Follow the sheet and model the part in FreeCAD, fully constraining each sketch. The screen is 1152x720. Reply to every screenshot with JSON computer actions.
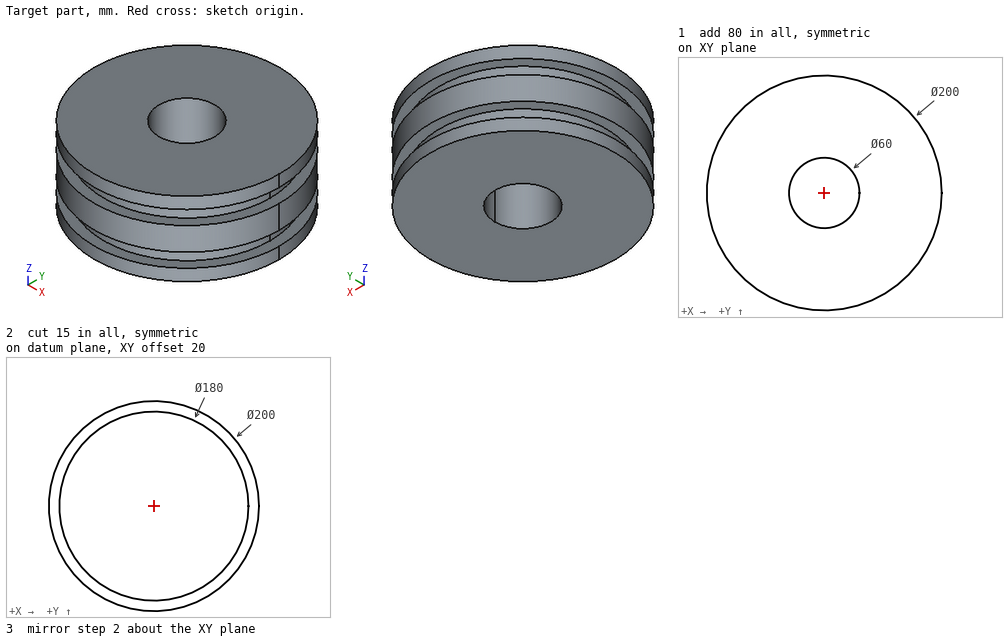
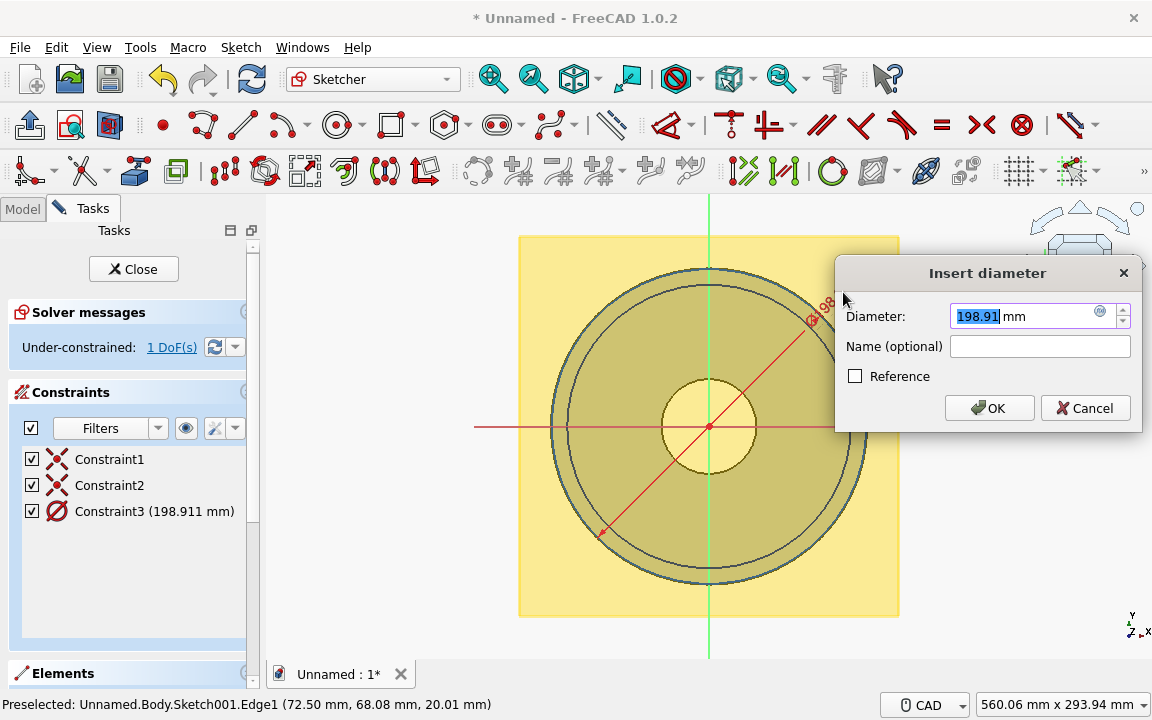
{"action": "type", "text": "200"}
{"action": "key", "text": "Return"}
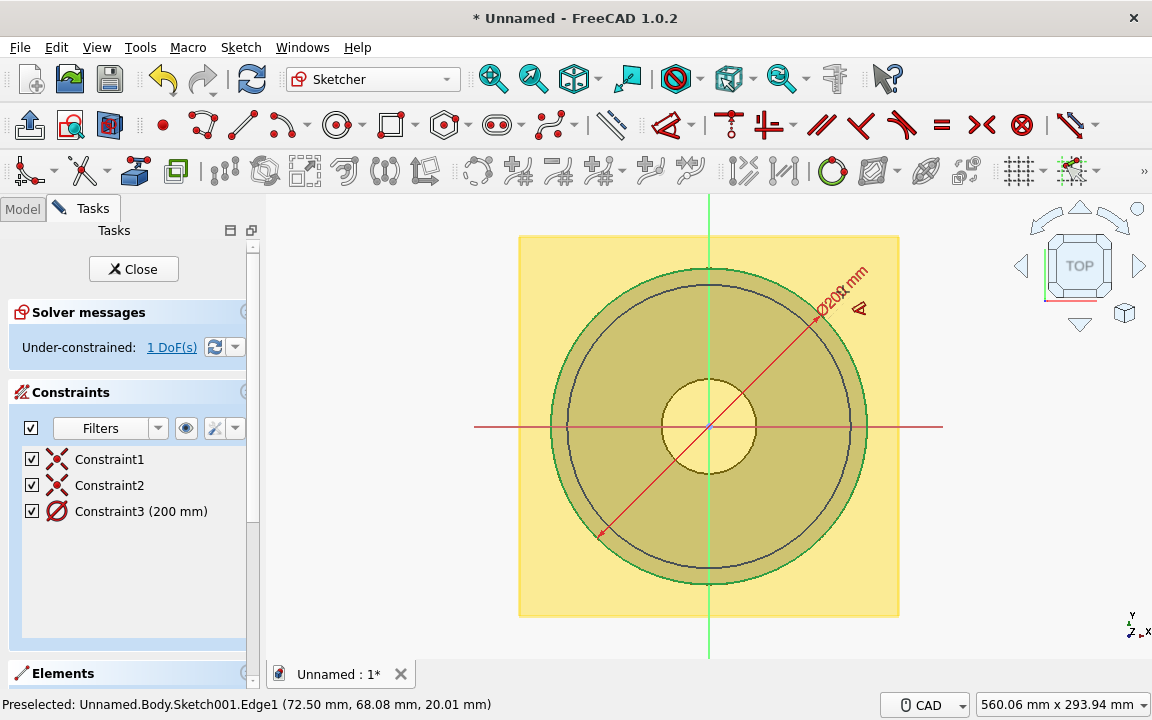
{"action": "left_click", "coordinate": [809, 326]}
{"action": "left_click", "coordinate": [876, 377]}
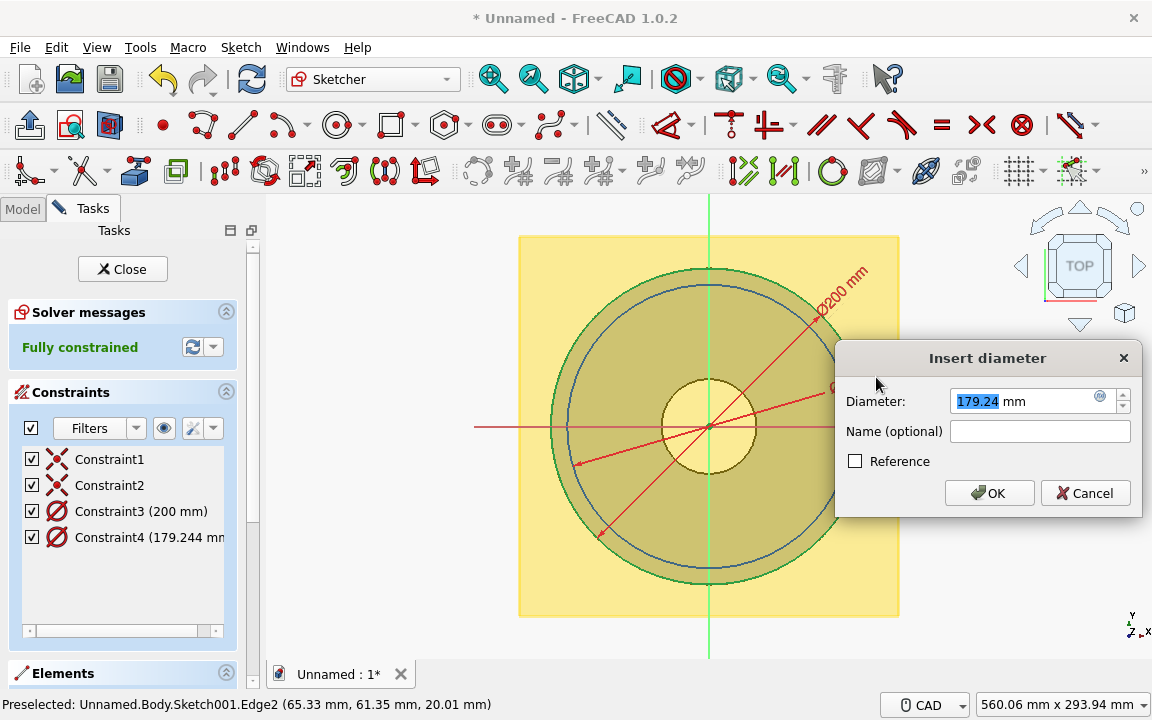
{"action": "type", "text": "180"}
{"action": "key", "text": "Return"}
{"action": "key", "text": "Escape"}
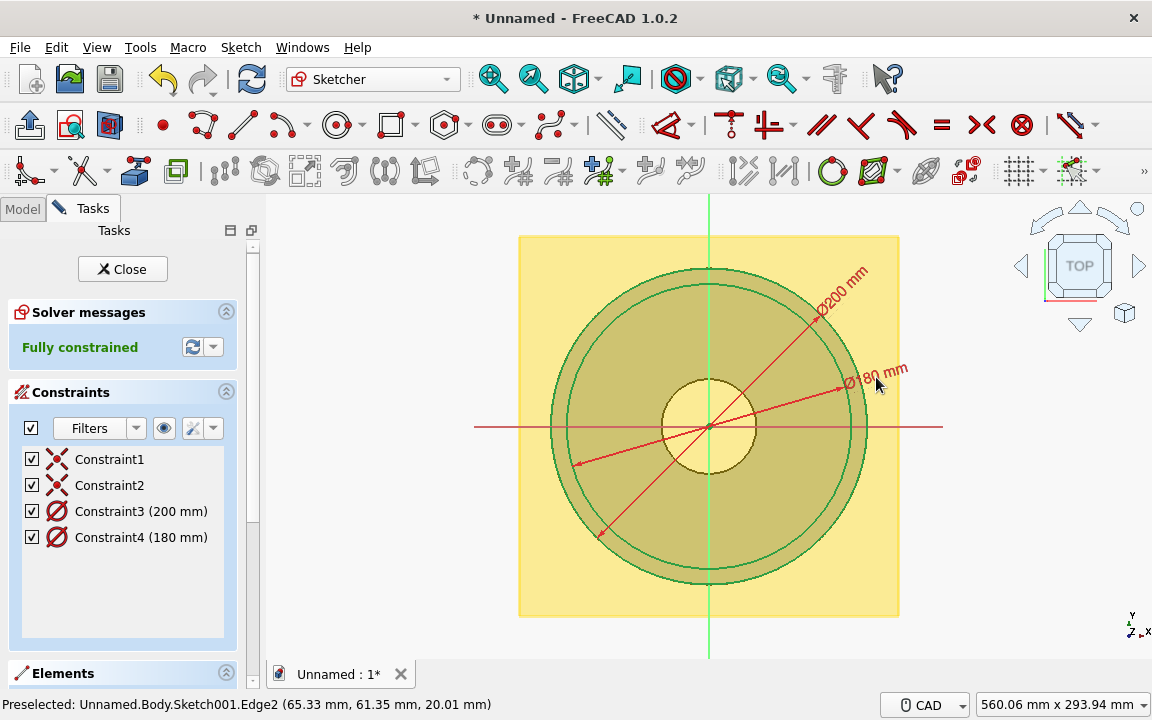
{"action": "left_click", "coordinate": [123, 269]}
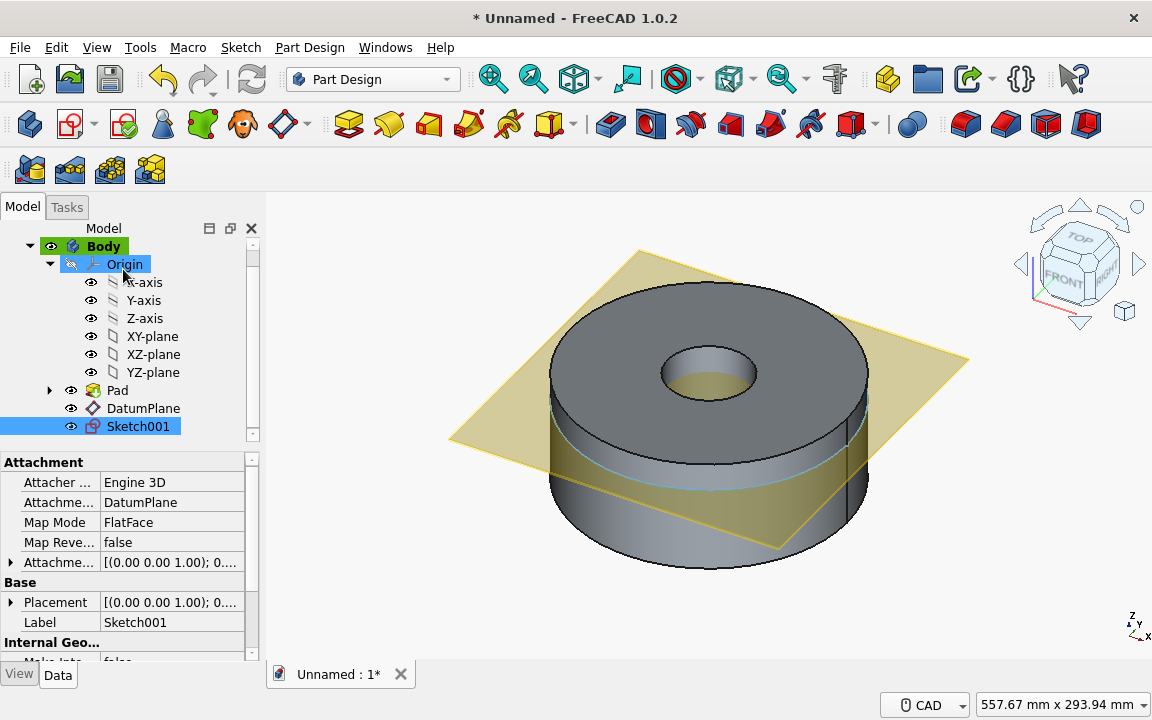
{"action": "left_click", "coordinate": [612, 124]}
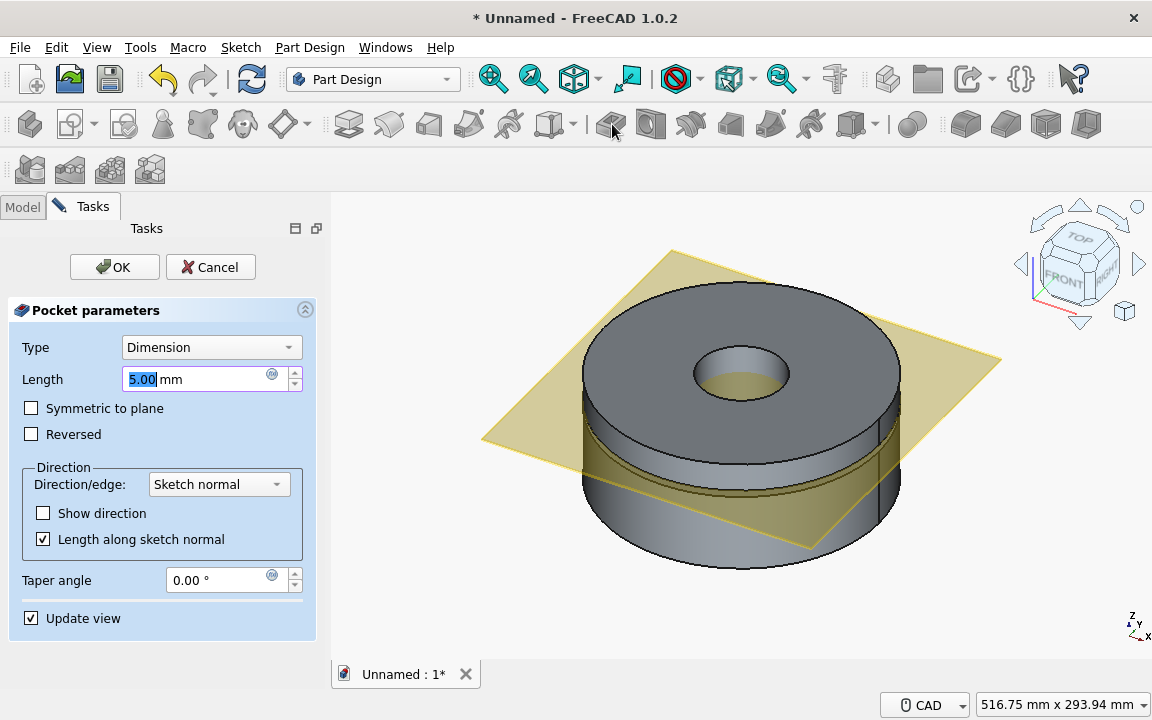
{"action": "type", "text": "15"}
{"action": "key", "text": "Tab"}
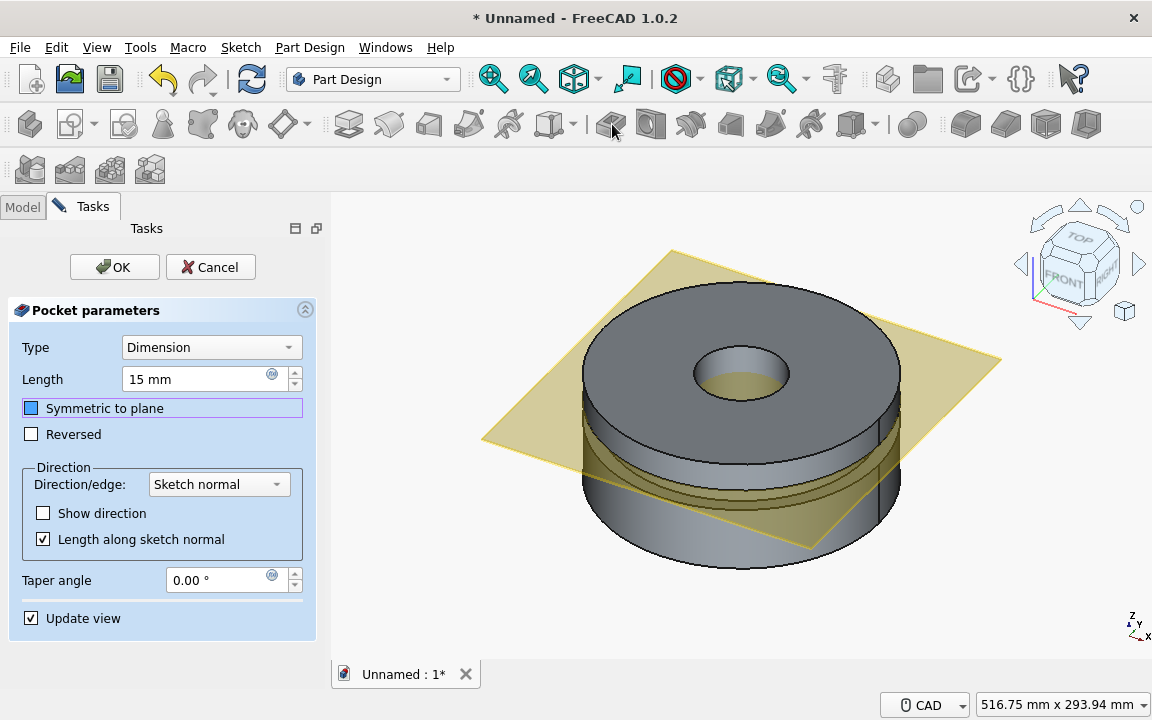
{"action": "left_click", "coordinate": [30, 408]}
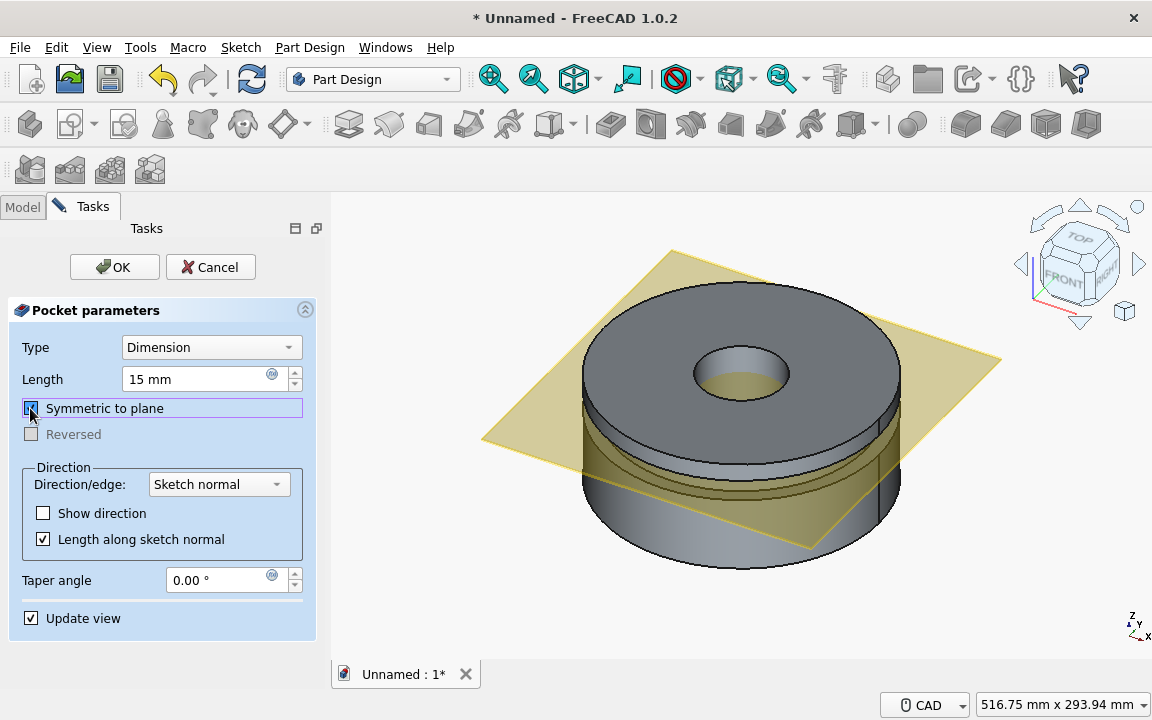
{"action": "left_click", "coordinate": [115, 267]}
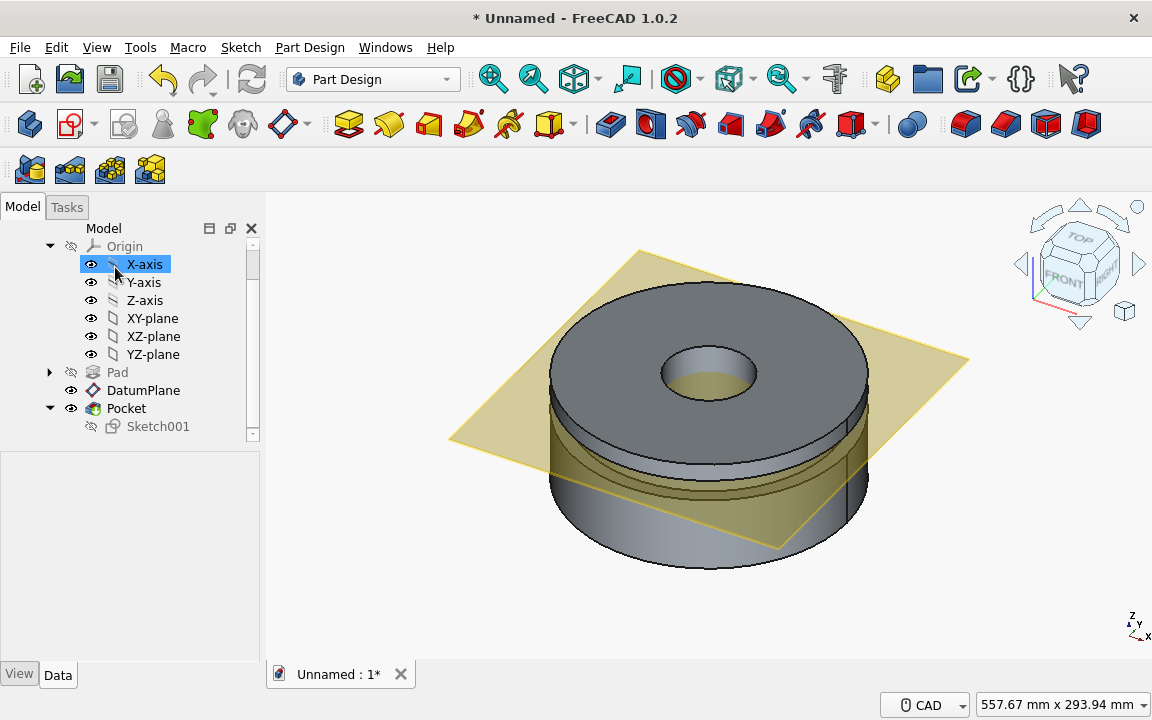
{"action": "left_click", "coordinate": [116, 390]}
{"action": "key", "text": "space"}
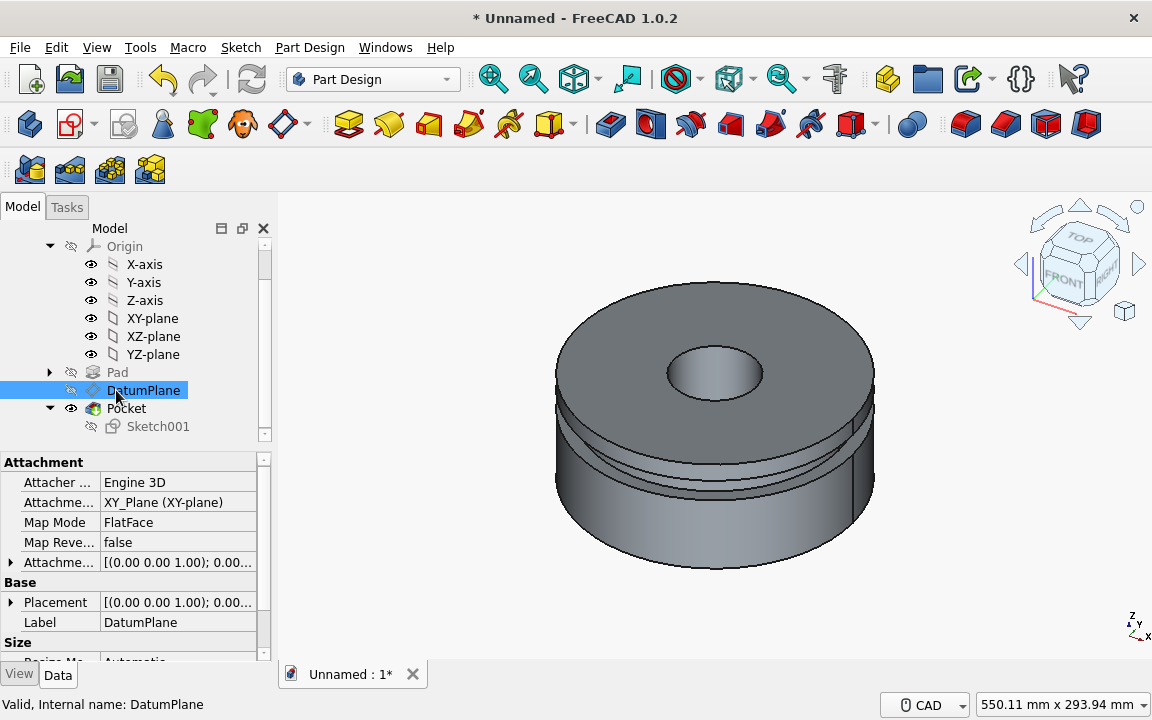
{"action": "left_click", "coordinate": [116, 408]}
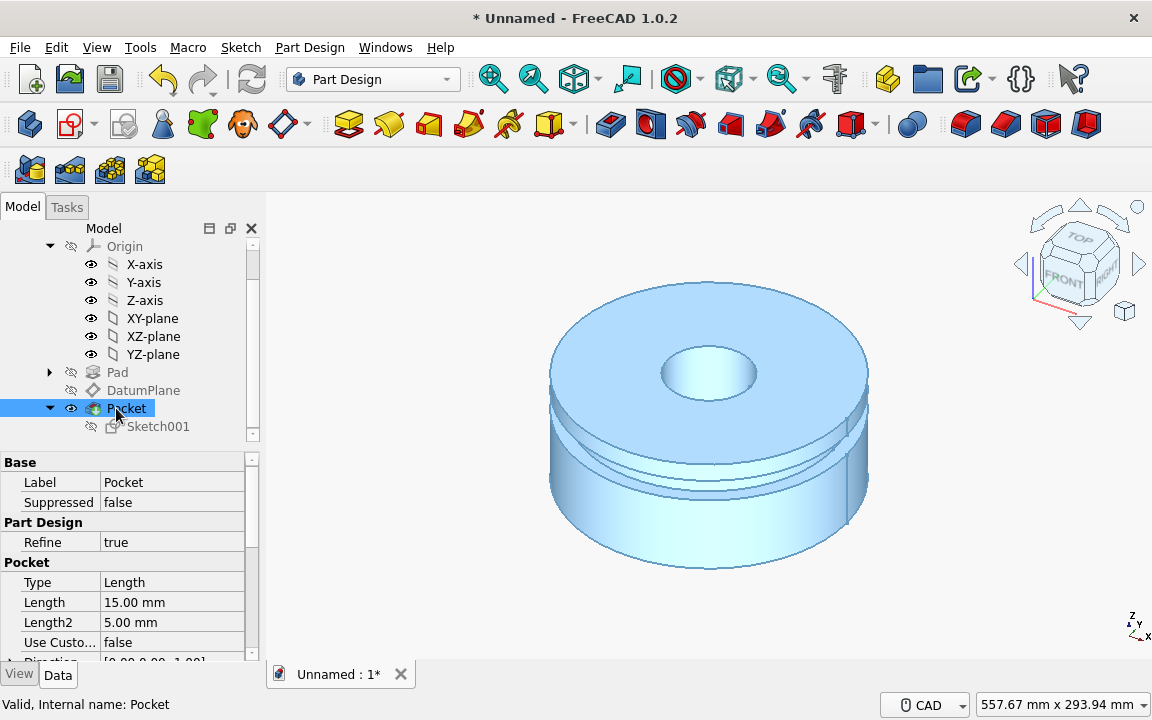
{"action": "left_click", "coordinate": [30, 170]}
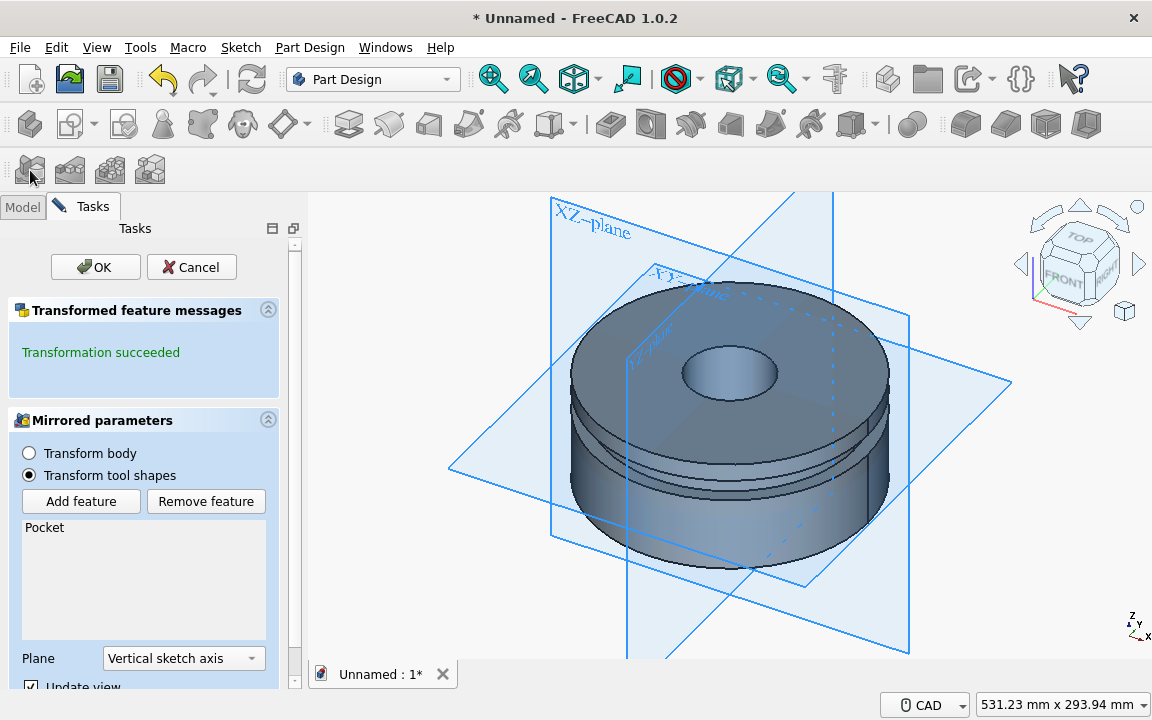
{"action": "left_click", "coordinate": [184, 658]}